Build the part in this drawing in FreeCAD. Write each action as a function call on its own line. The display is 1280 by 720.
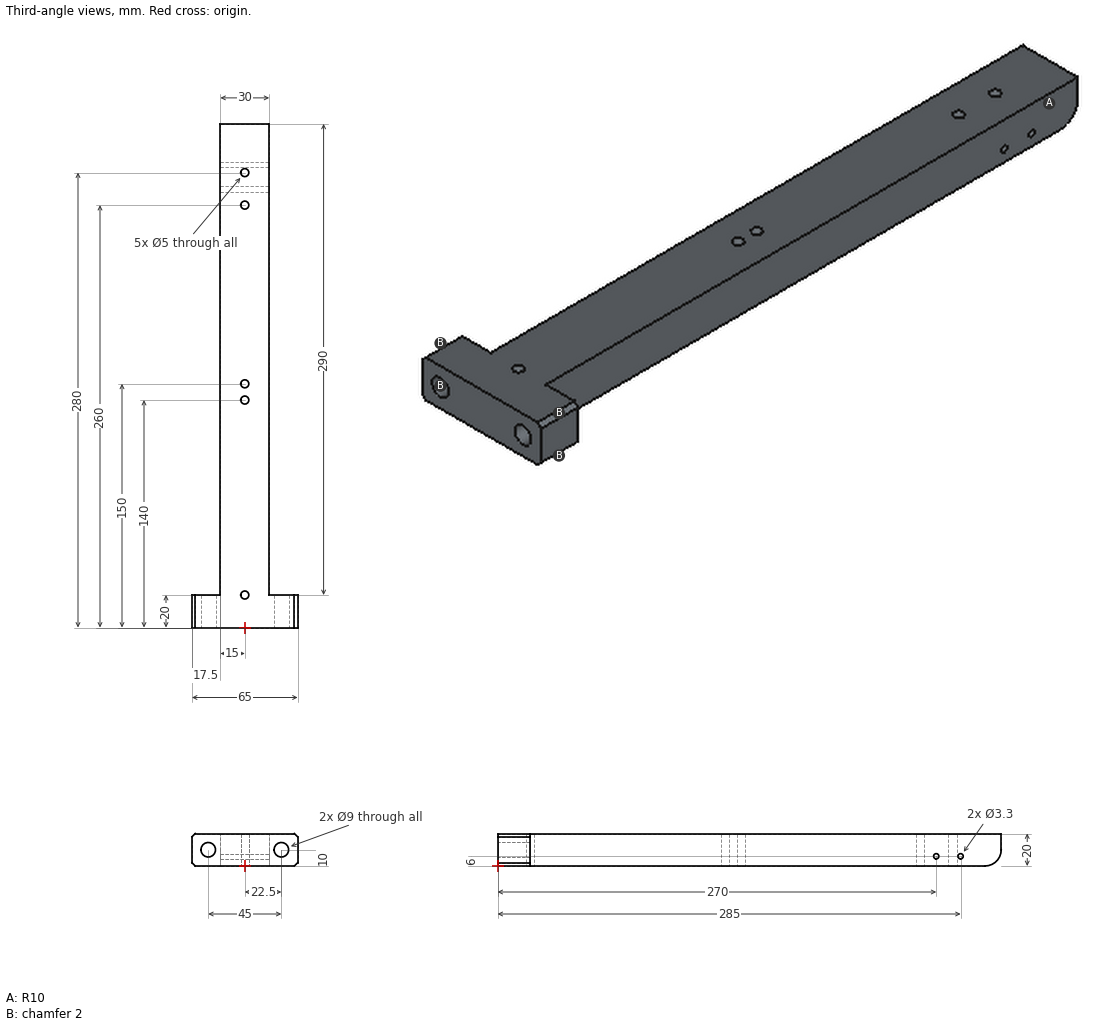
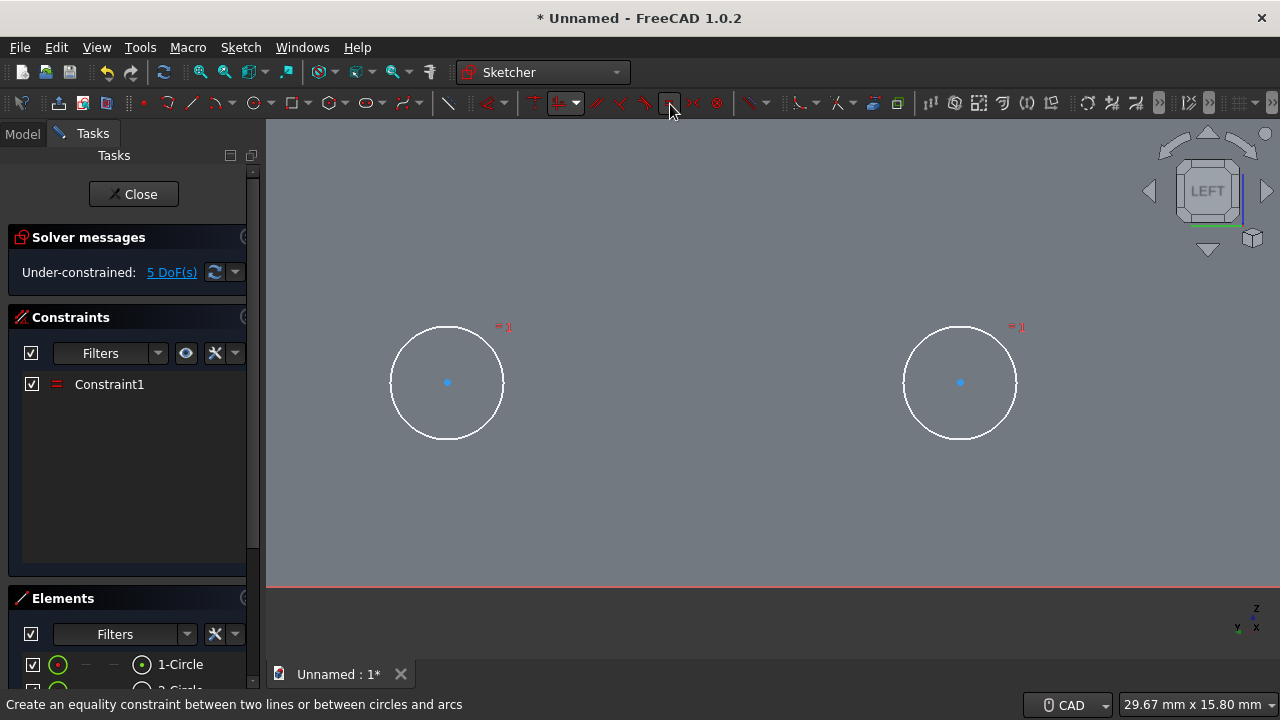
click(447, 383)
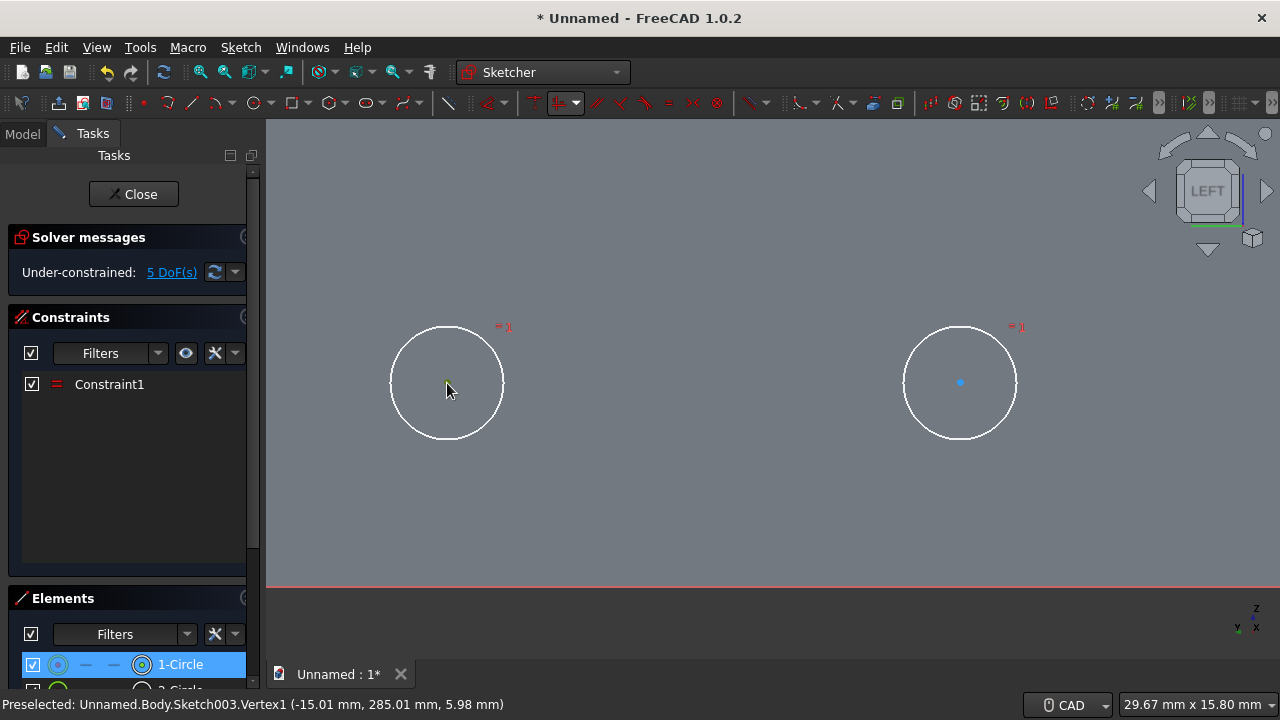
click(960, 383)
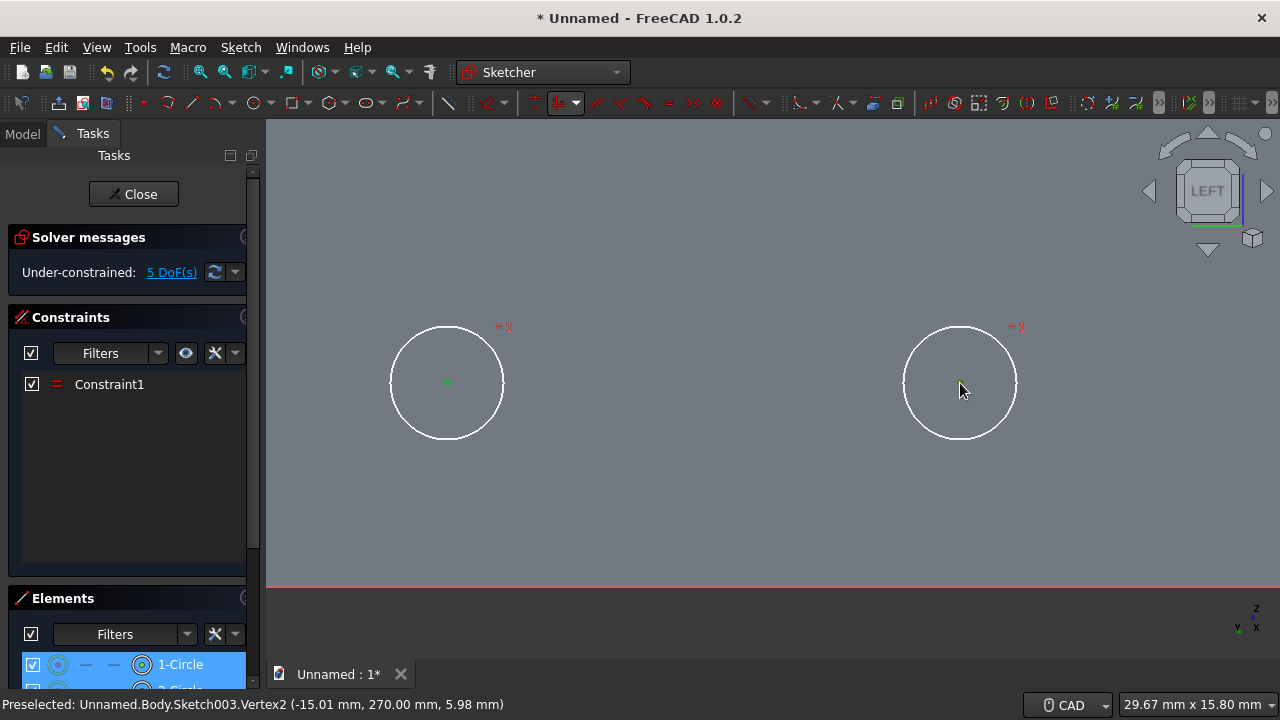
key(h)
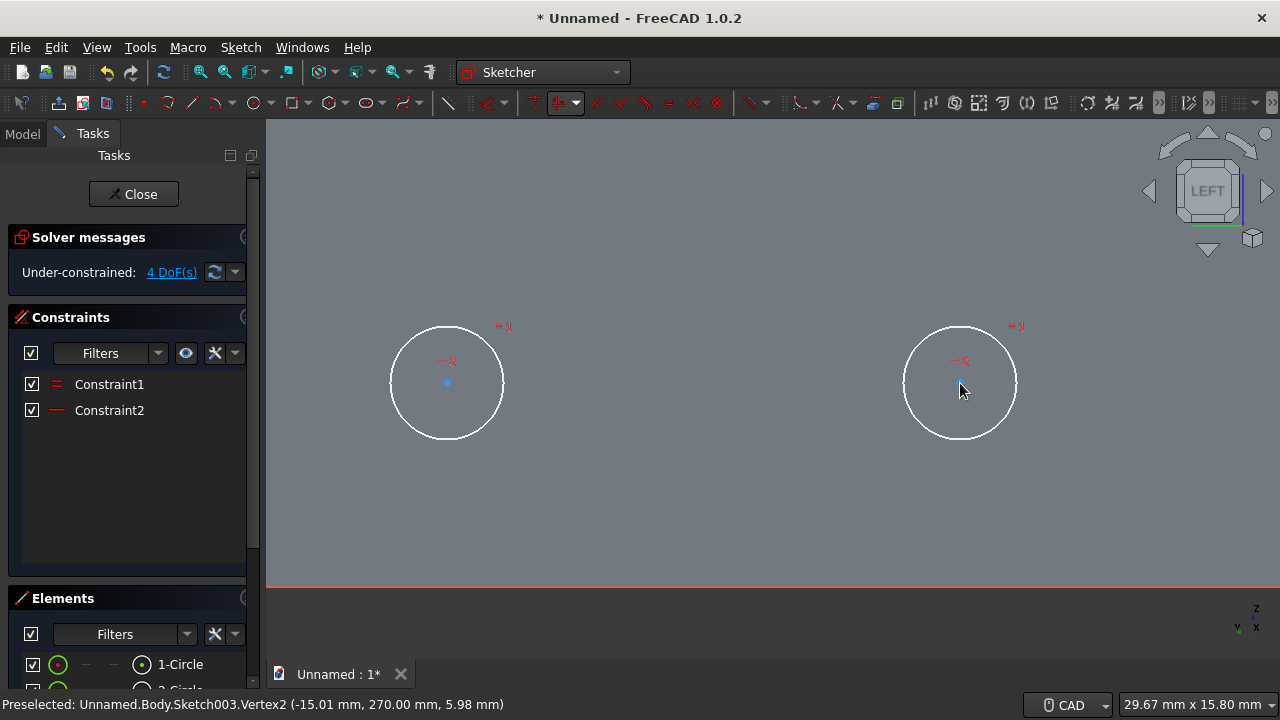
click(488, 104)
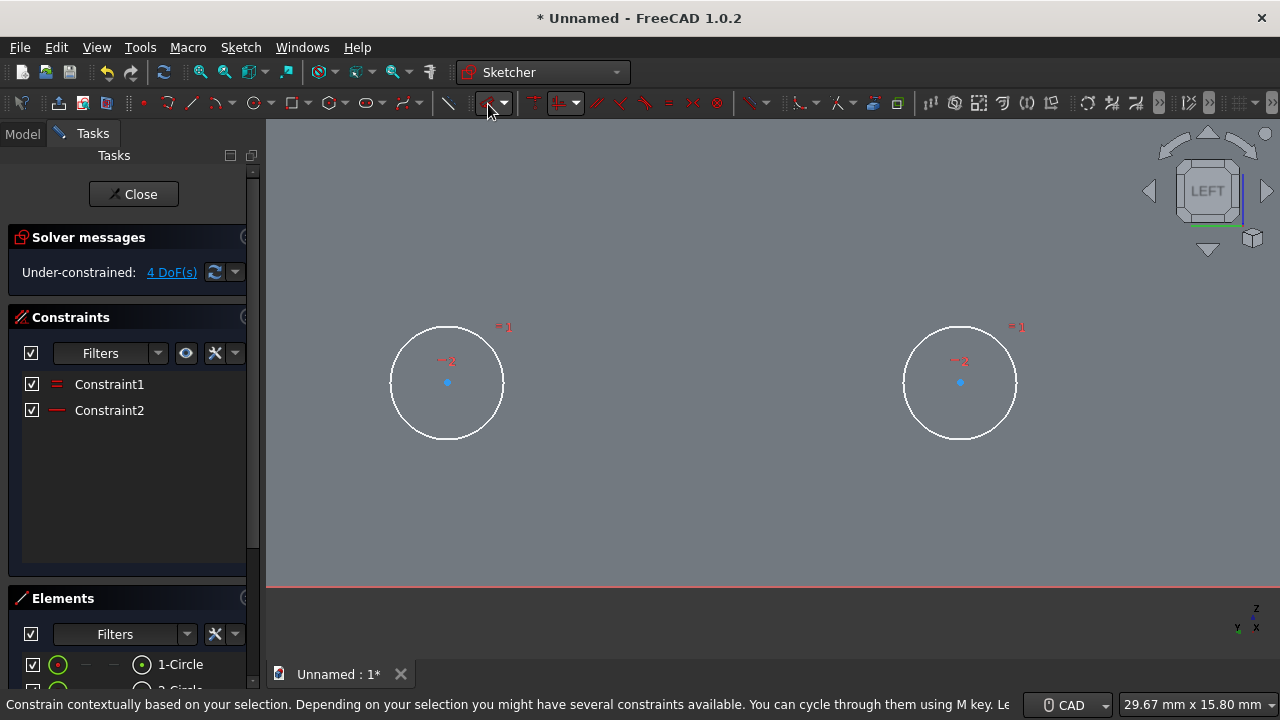
click(487, 343)
click(510, 320)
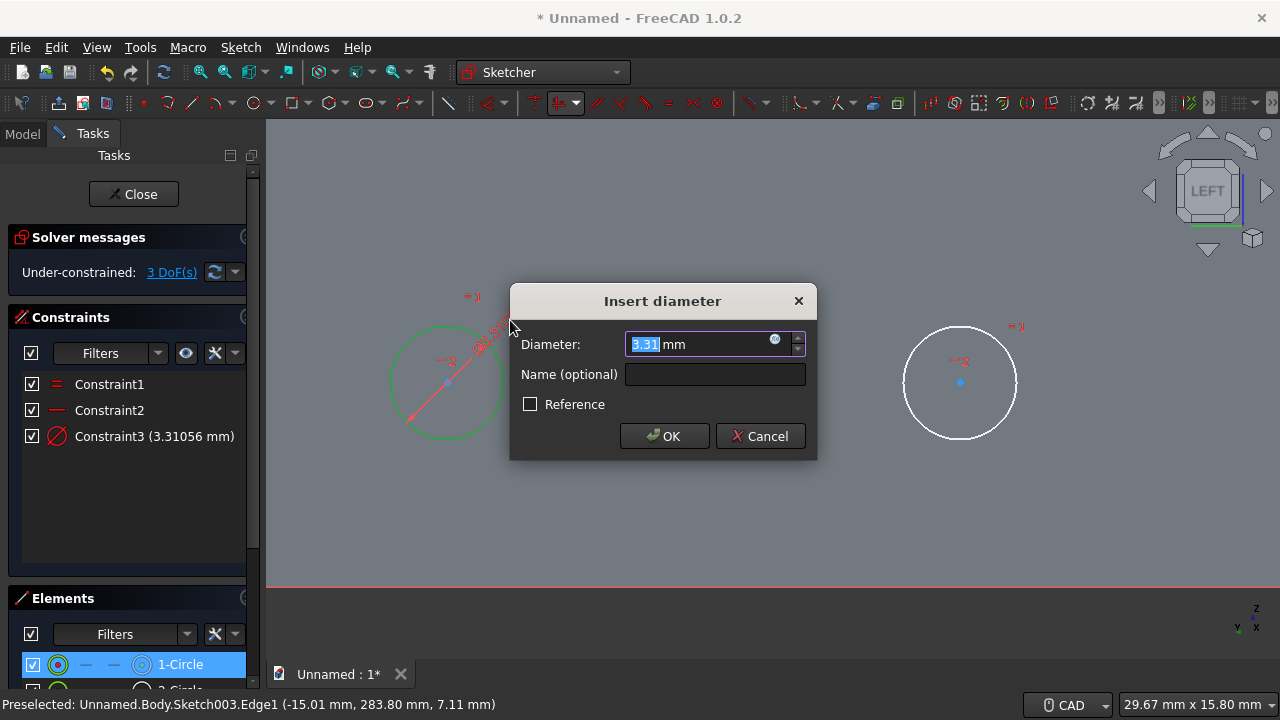
text(3.3)
key(Return)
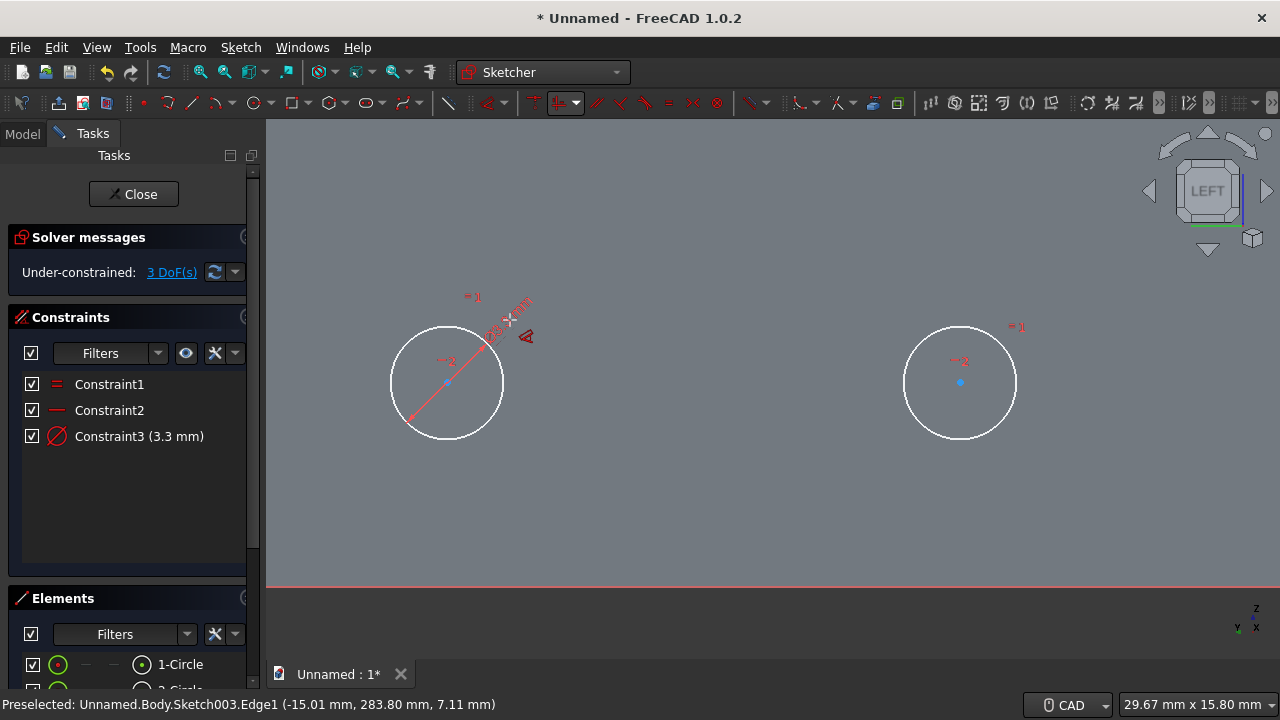
click(447, 383)
click(413, 485)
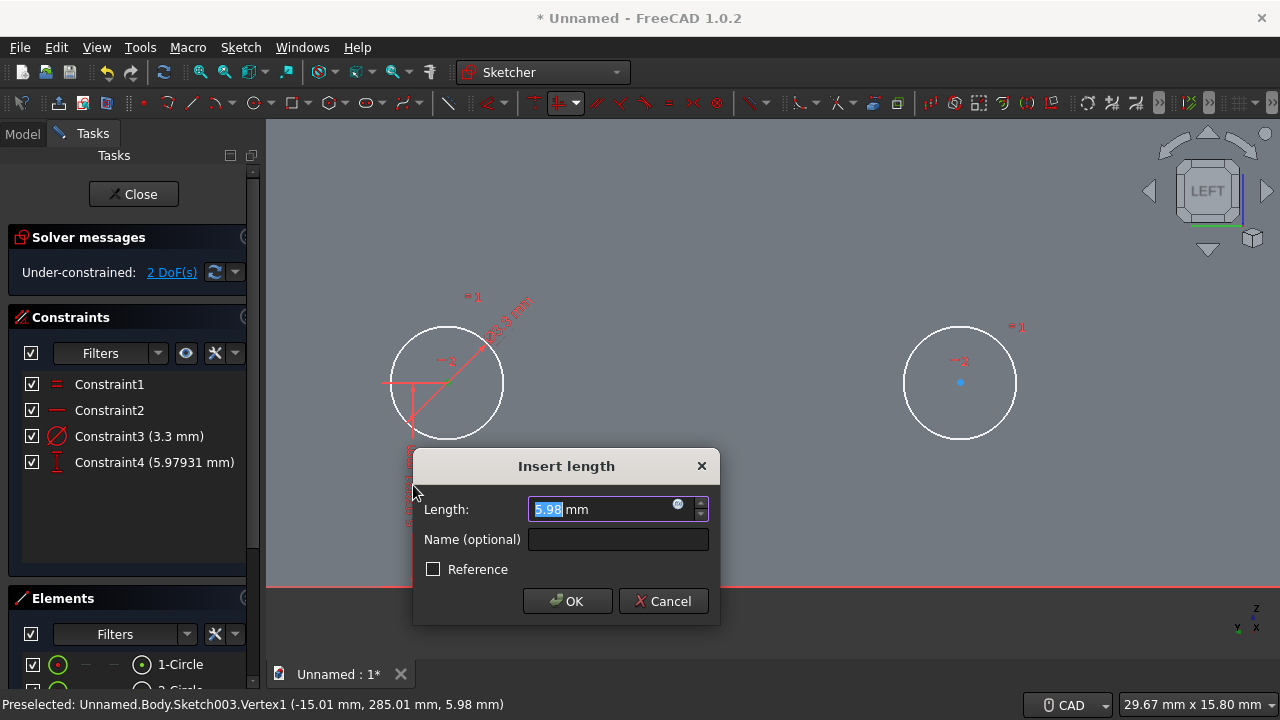
text(6)
key(Return)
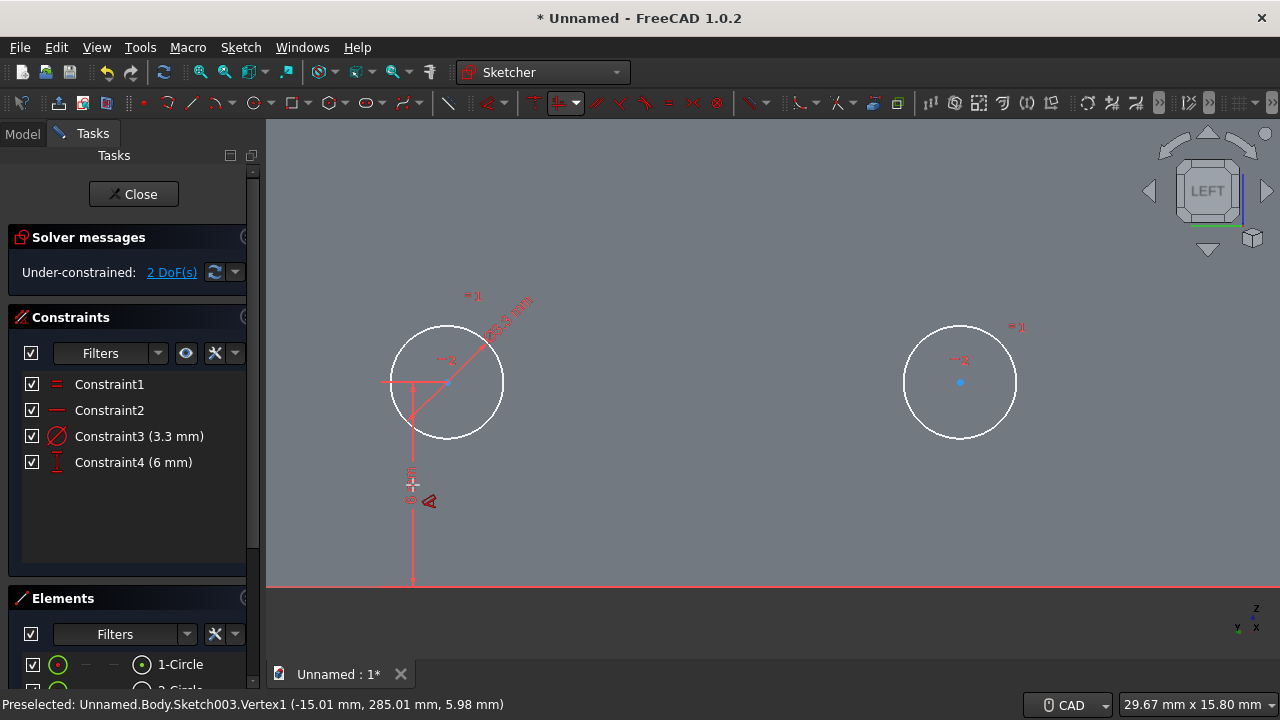
click(447, 382)
click(781, 621)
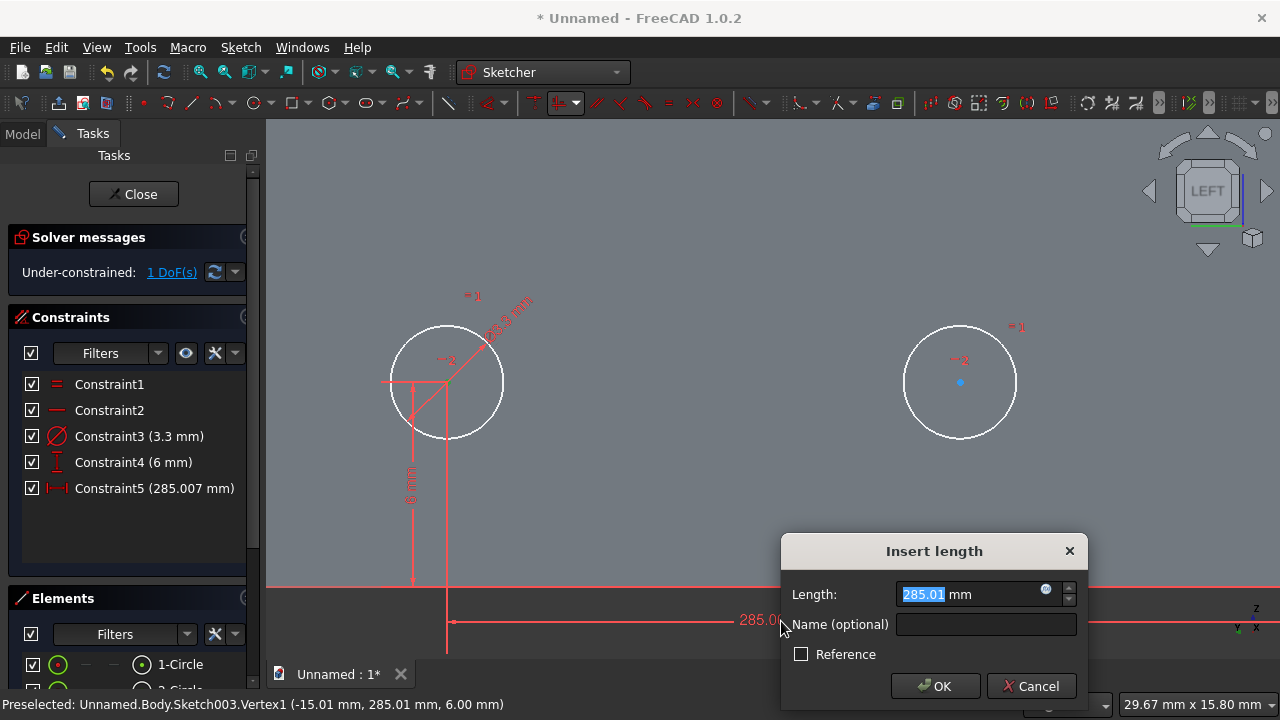
text(285)
key(Return)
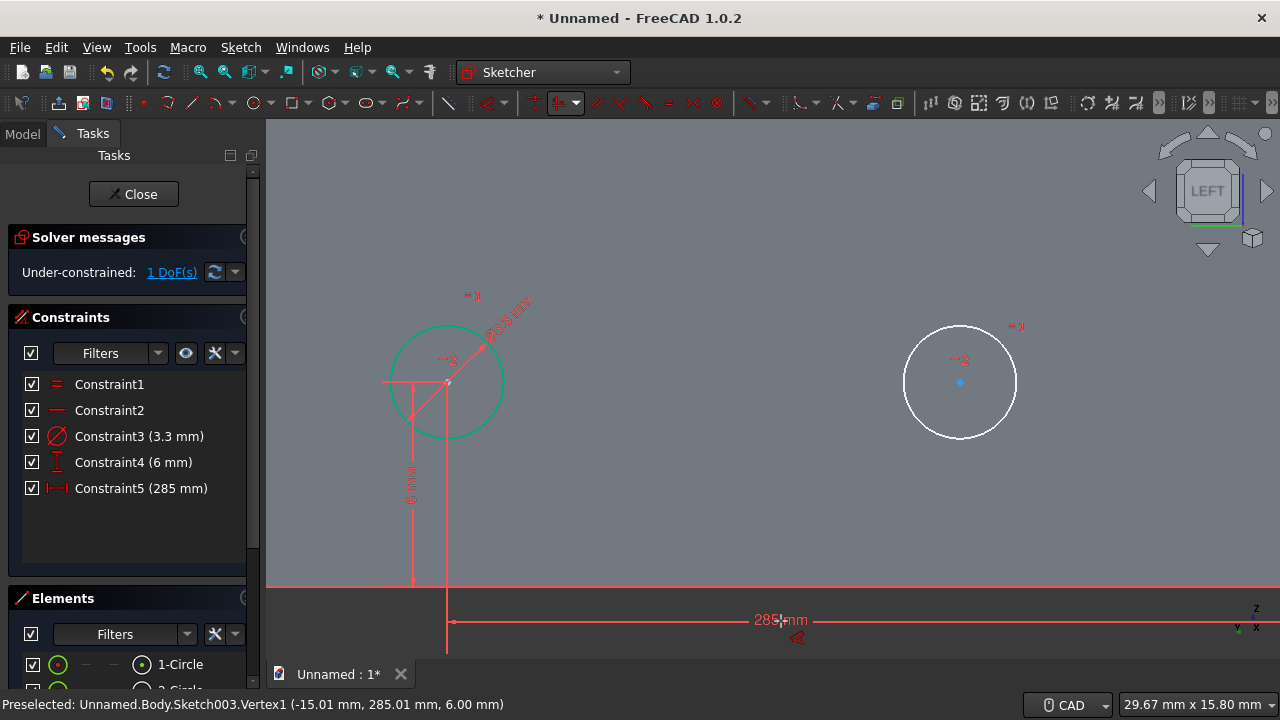
click(960, 382)
click(1037, 621)